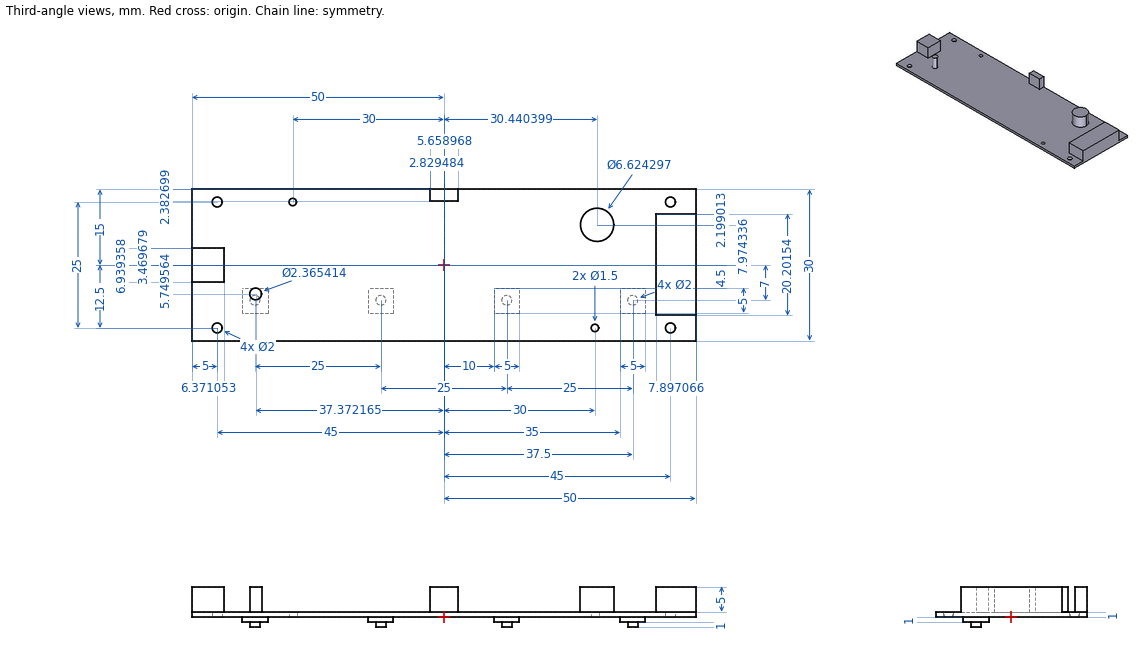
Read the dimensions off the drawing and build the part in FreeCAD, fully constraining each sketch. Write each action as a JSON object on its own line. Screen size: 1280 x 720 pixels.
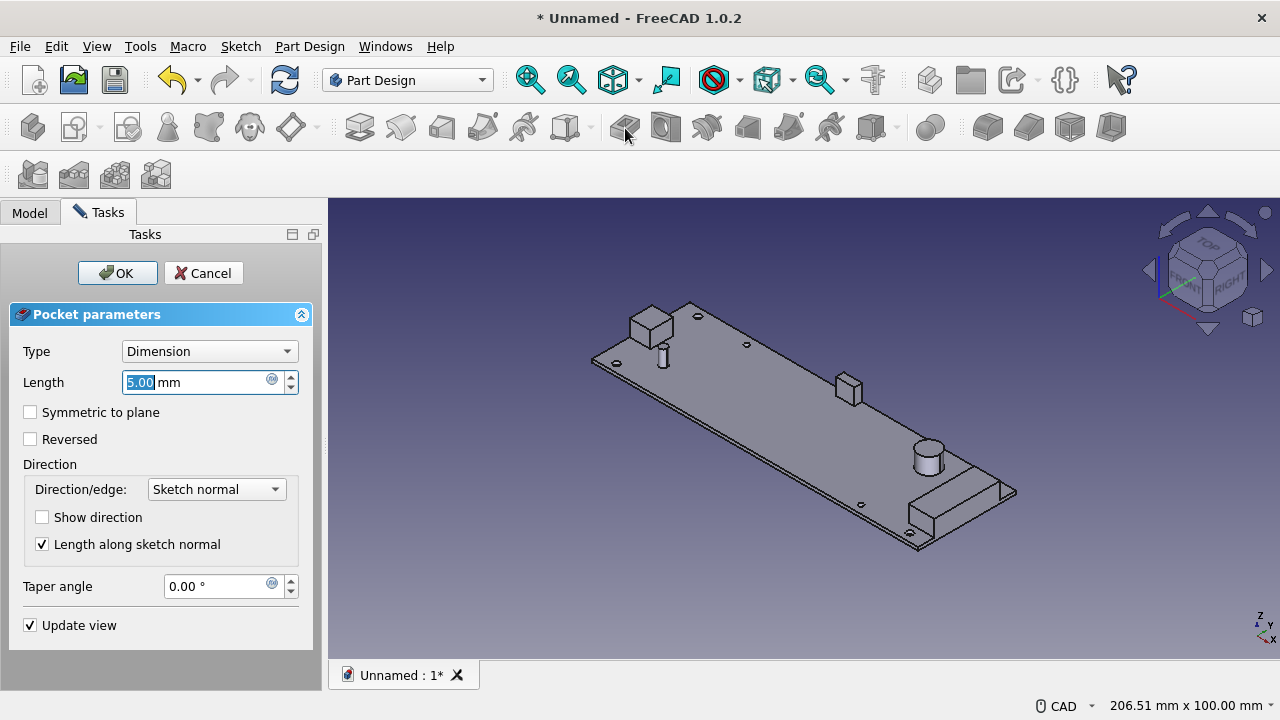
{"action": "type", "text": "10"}
{"action": "key", "text": "Tab"}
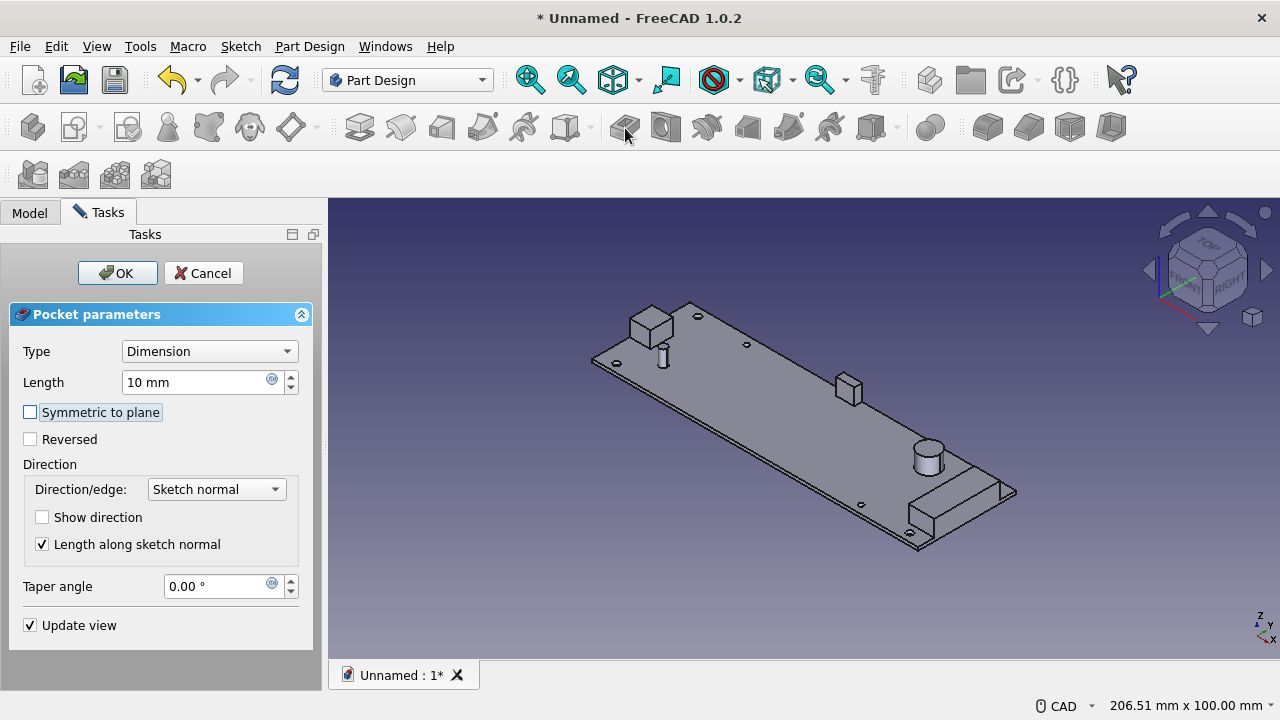
{"action": "left_click", "coordinate": [118, 273]}